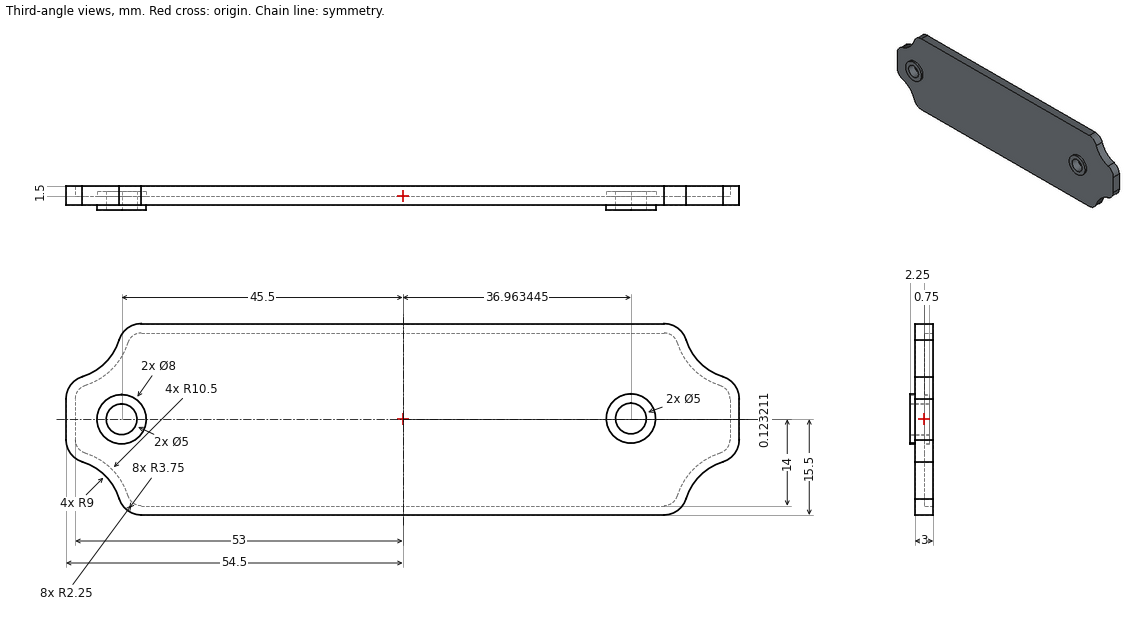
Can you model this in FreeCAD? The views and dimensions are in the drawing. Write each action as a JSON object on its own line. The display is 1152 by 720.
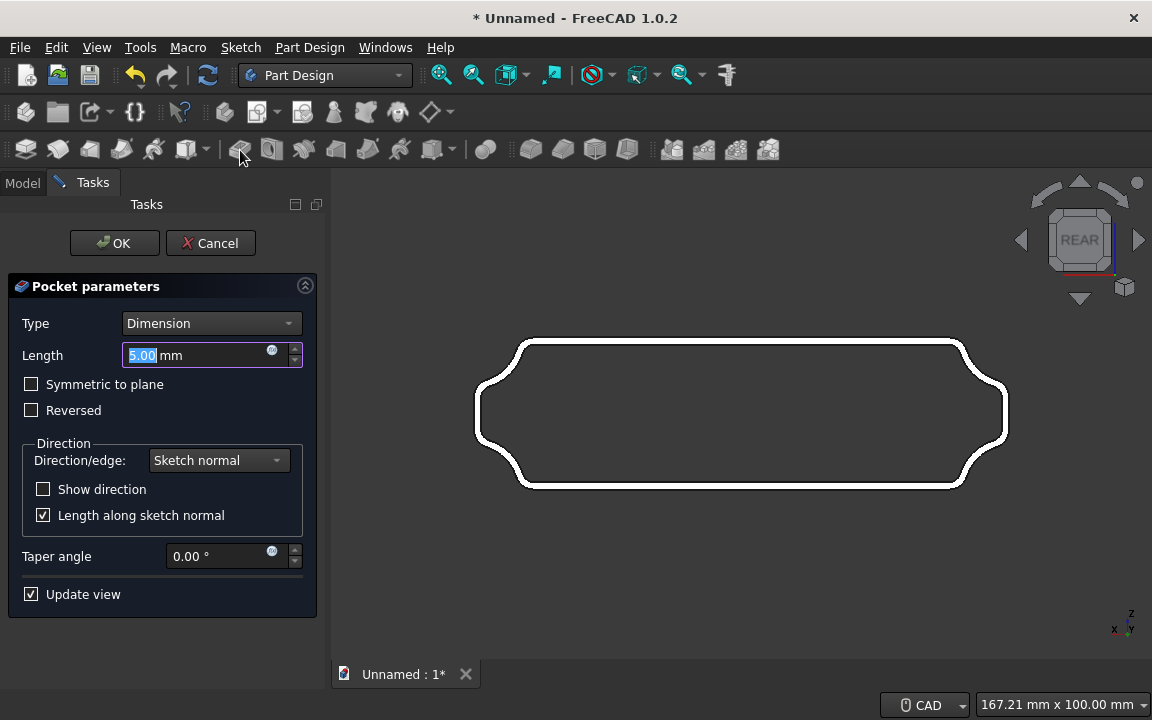
{"action": "type", "text": "1.5"}
{"action": "key", "text": "Tab"}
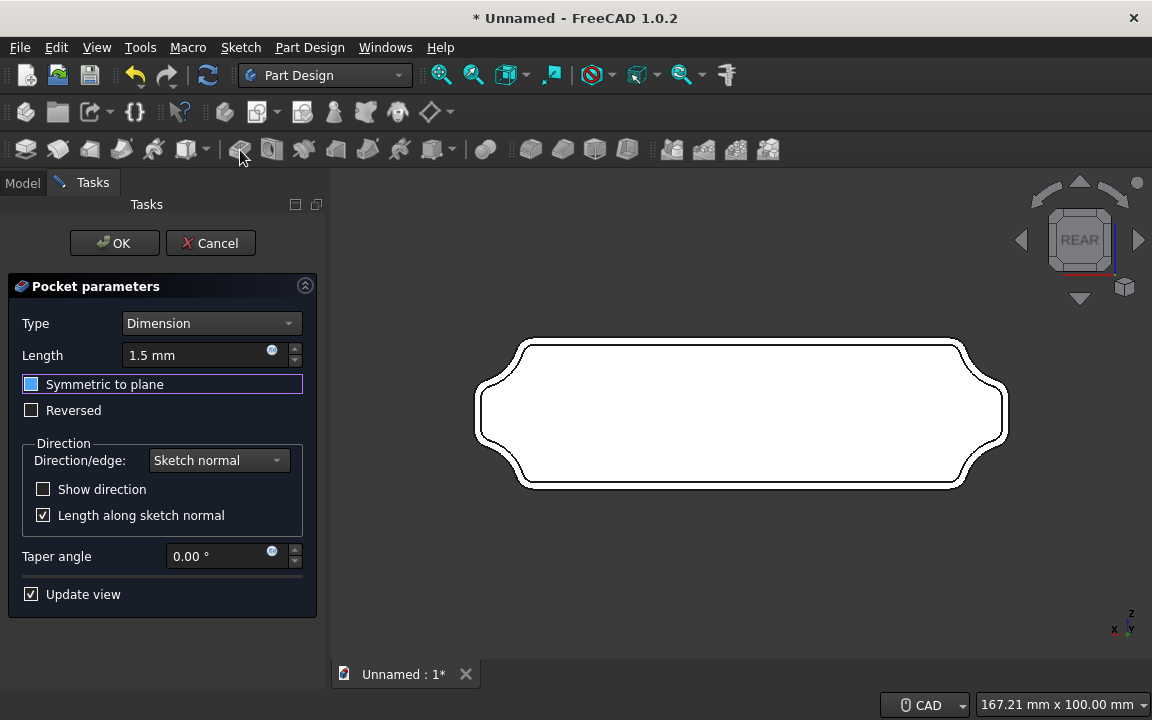
{"action": "left_click", "coordinate": [115, 243]}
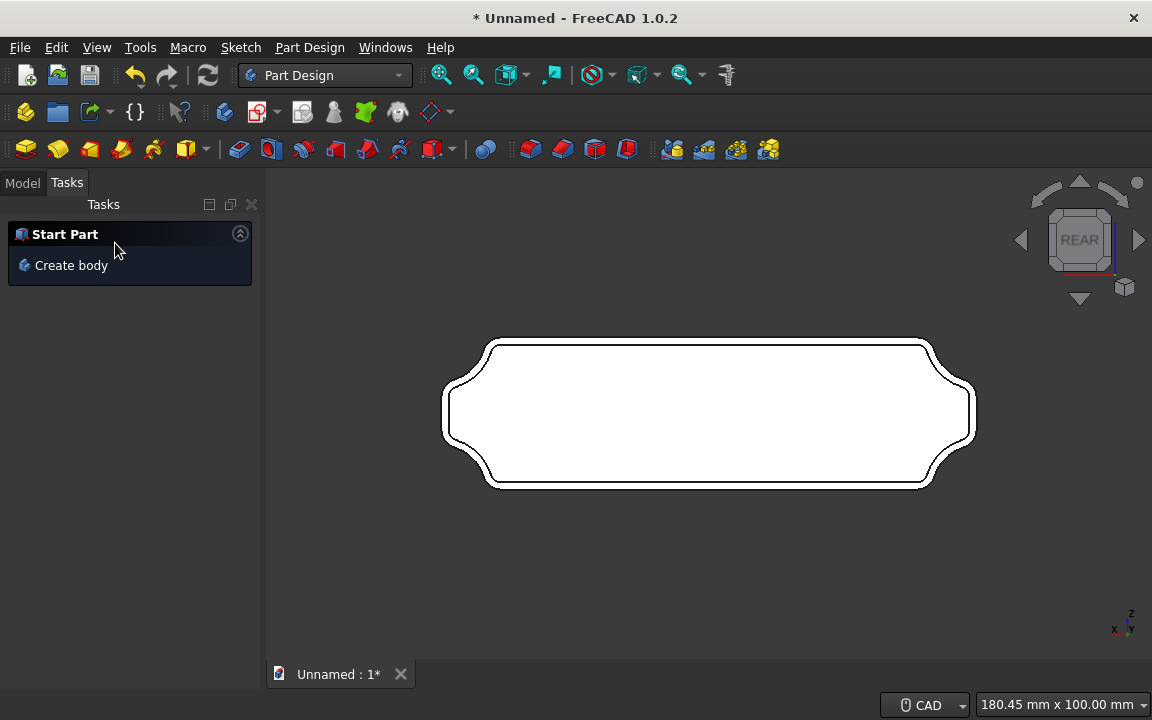
{"action": "left_click", "coordinate": [258, 112]}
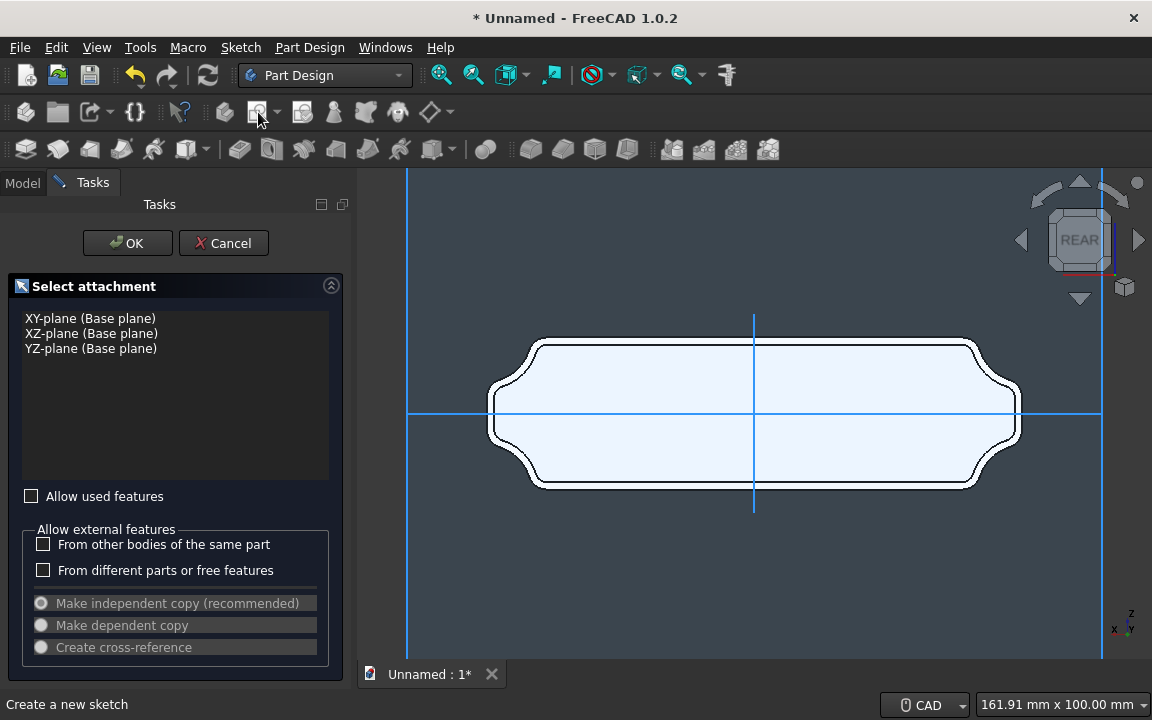
{"action": "left_click", "coordinate": [82, 334]}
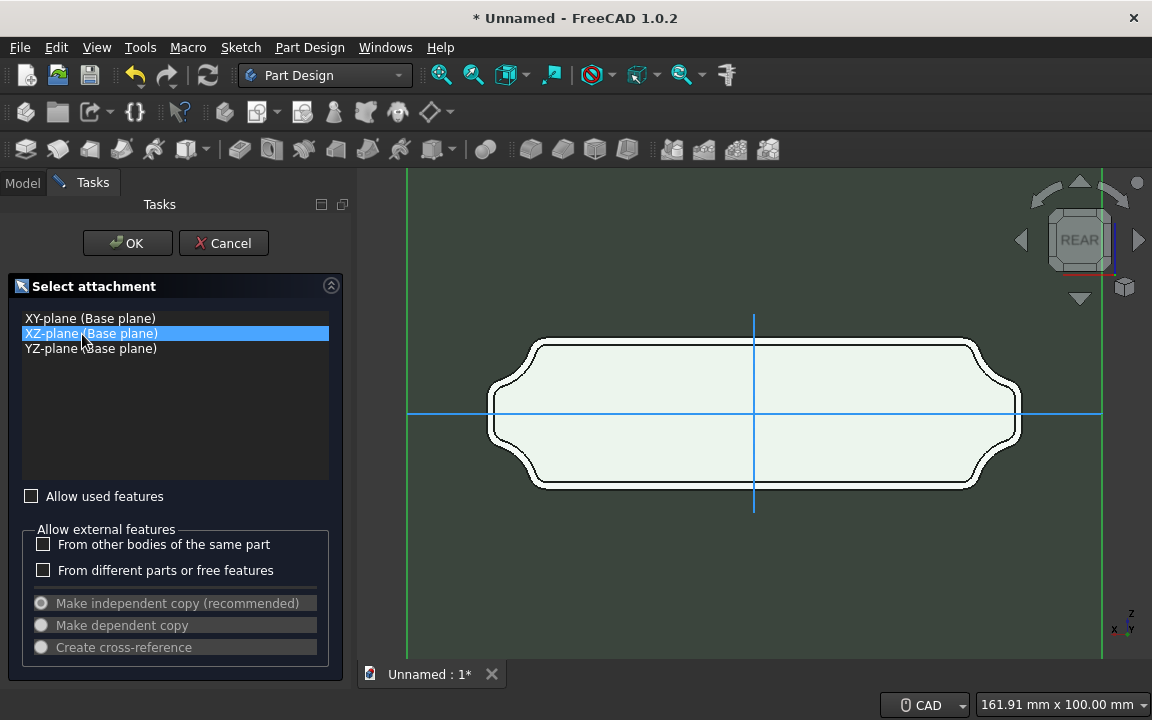
{"action": "left_click", "coordinate": [128, 243]}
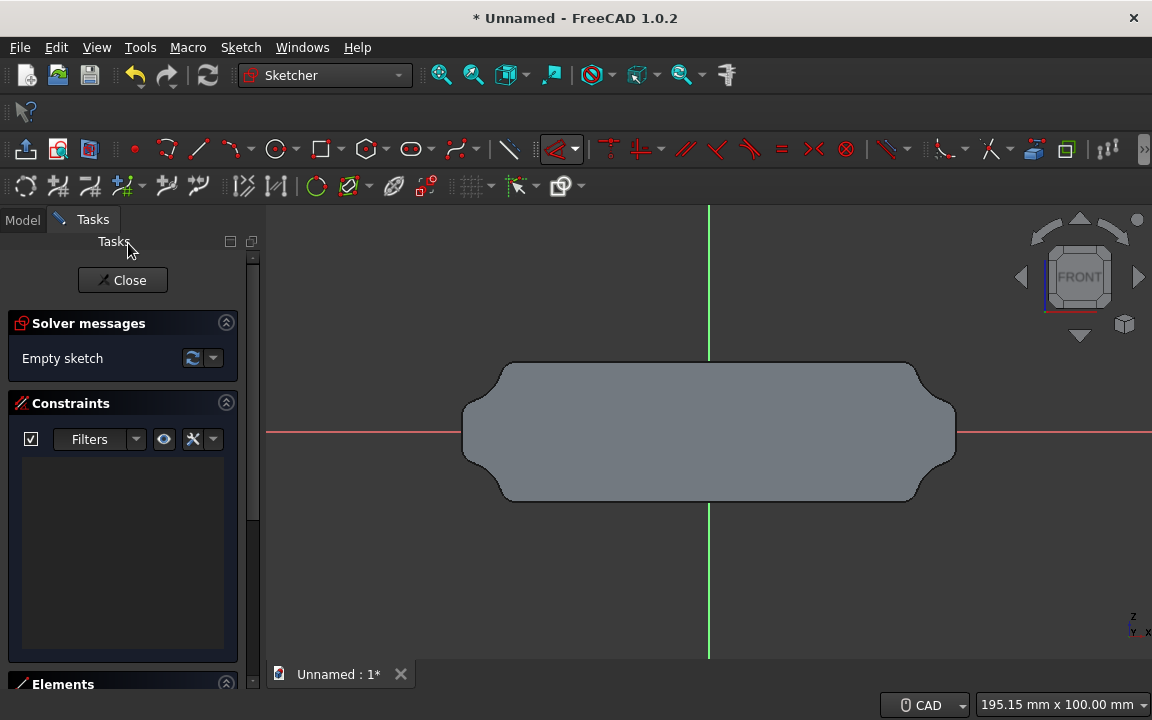
{"action": "left_click", "coordinate": [90, 150]}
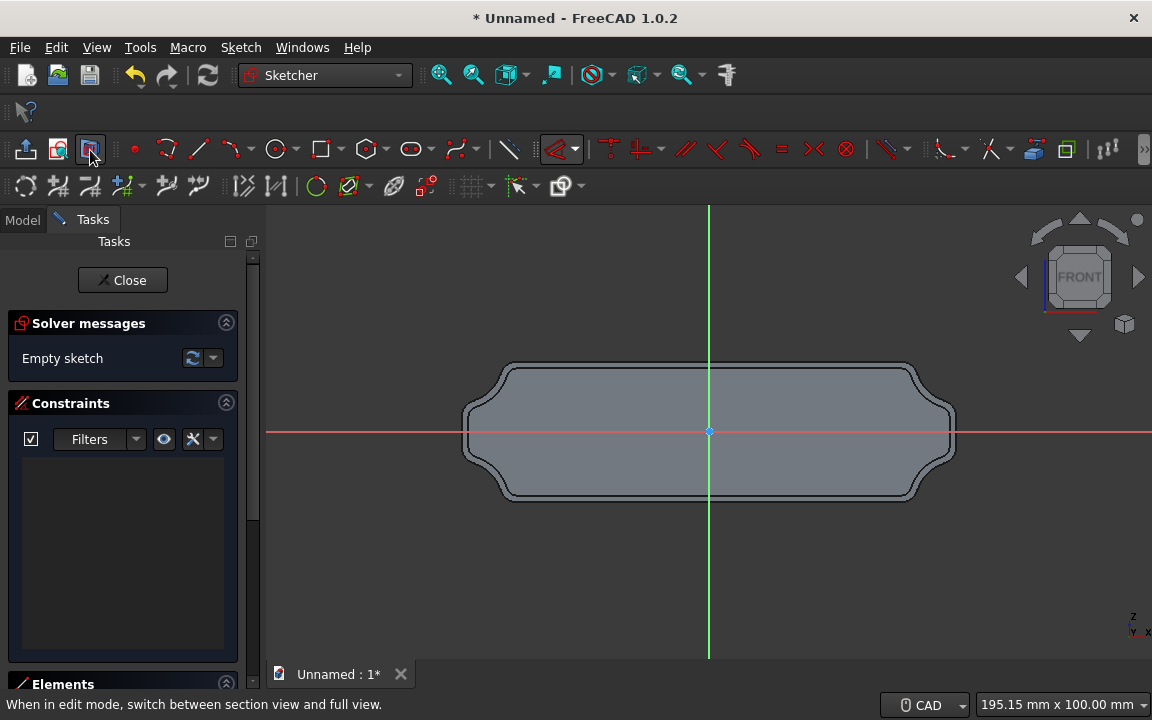
{"action": "left_click", "coordinate": [276, 150]}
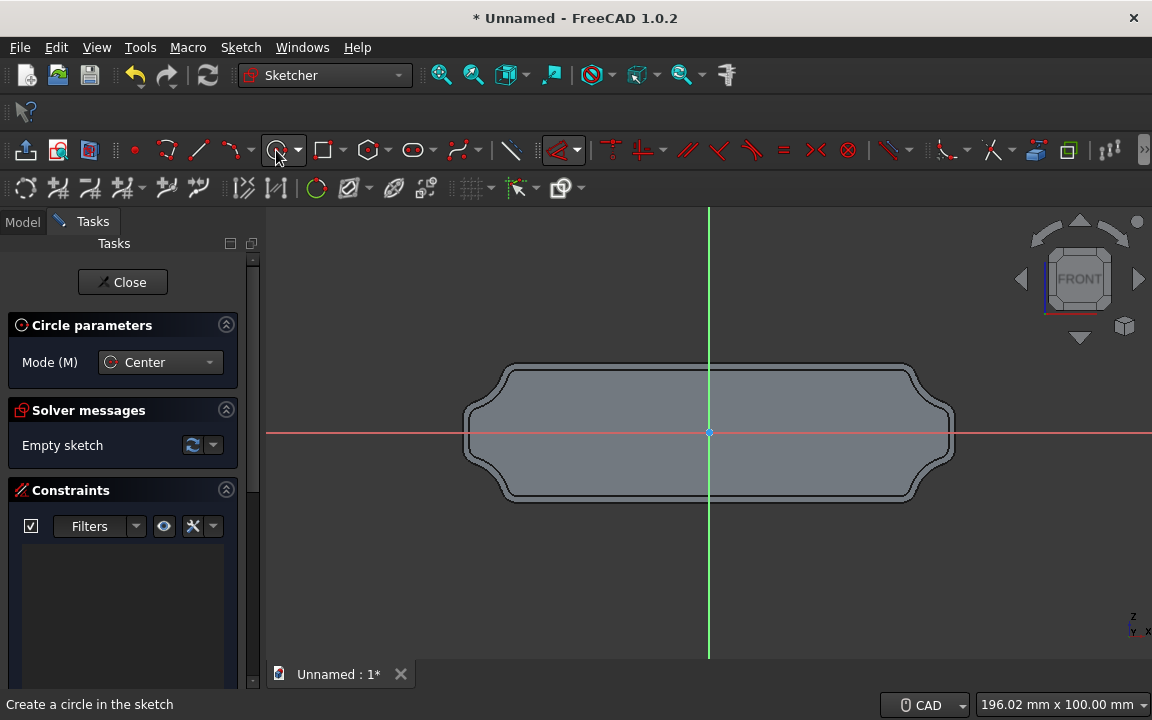
{"action": "scroll", "coordinate": [503, 433], "scroll_direction": "up", "scroll_amount": 2}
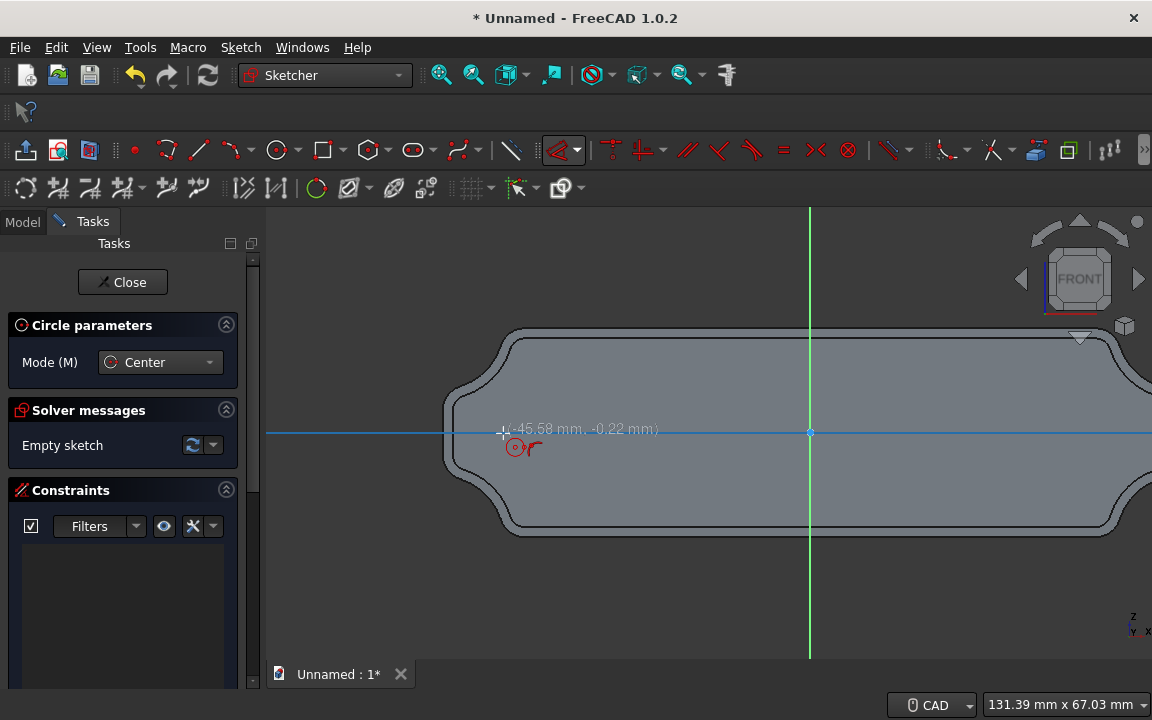
{"action": "left_click", "coordinate": [503, 433]}
{"action": "mouse_move", "coordinate": [522, 414]}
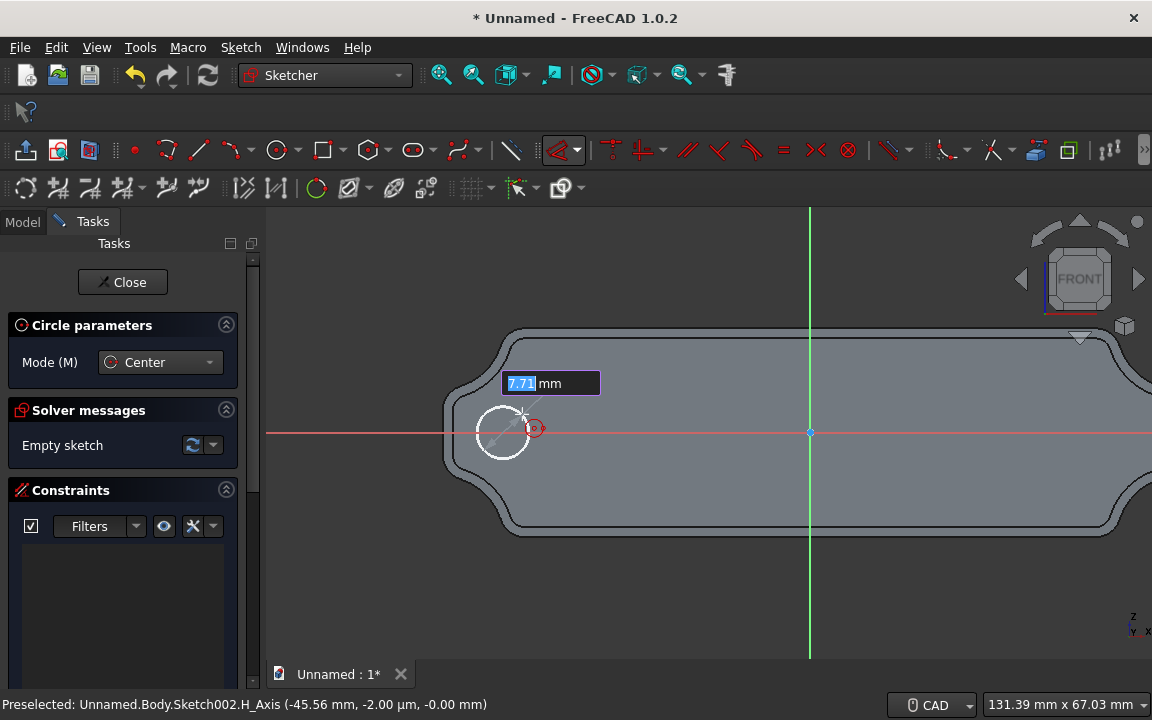
{"action": "type", "text": "8"}
{"action": "key", "text": "Return"}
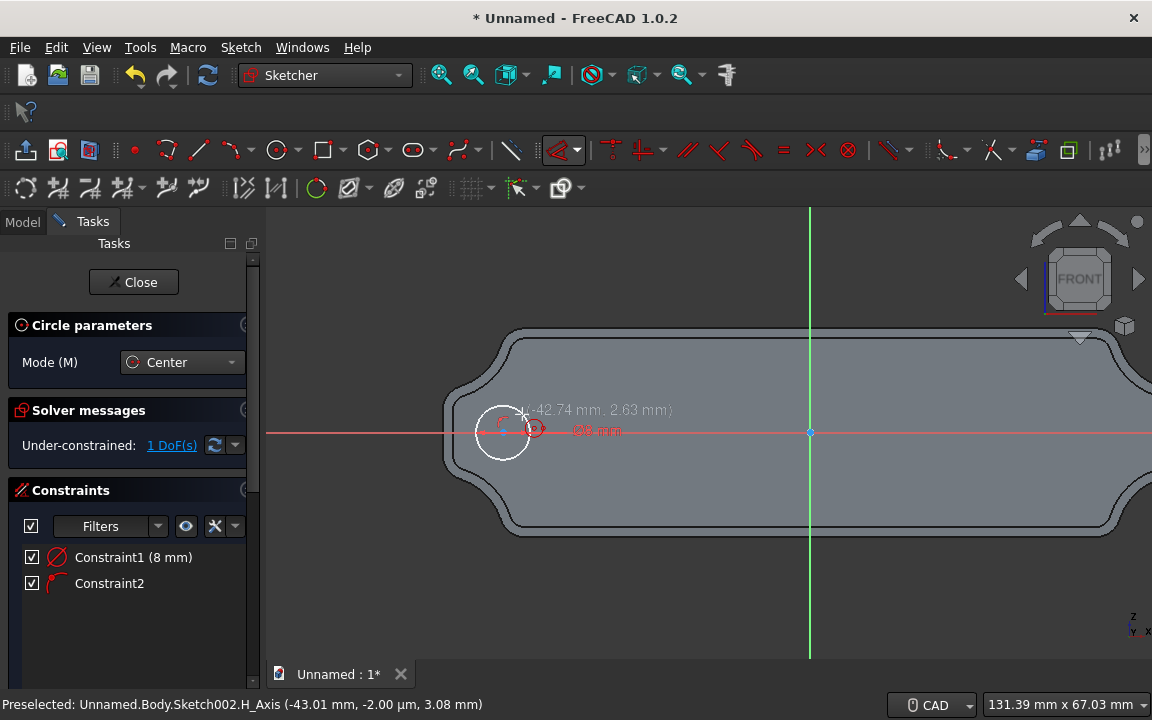
{"action": "scroll", "coordinate": [294, 436], "scroll_direction": "down", "scroll_amount": 1}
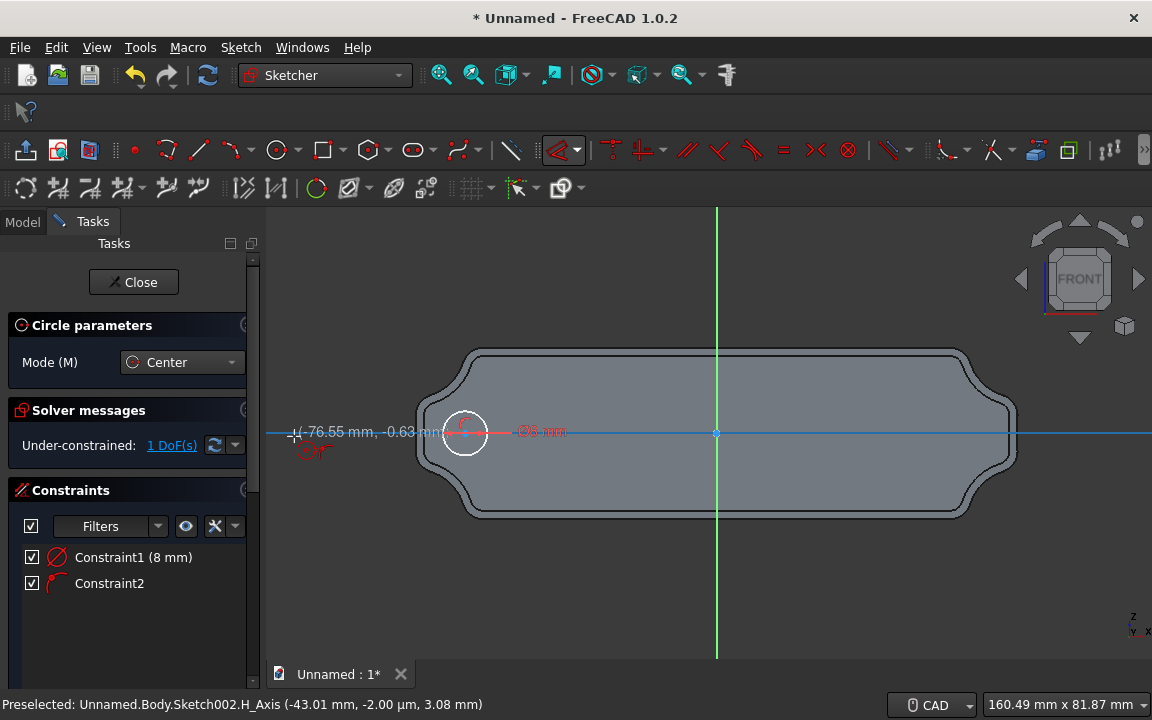
{"action": "scroll", "coordinate": [921, 433], "scroll_direction": "up", "scroll_amount": 16}